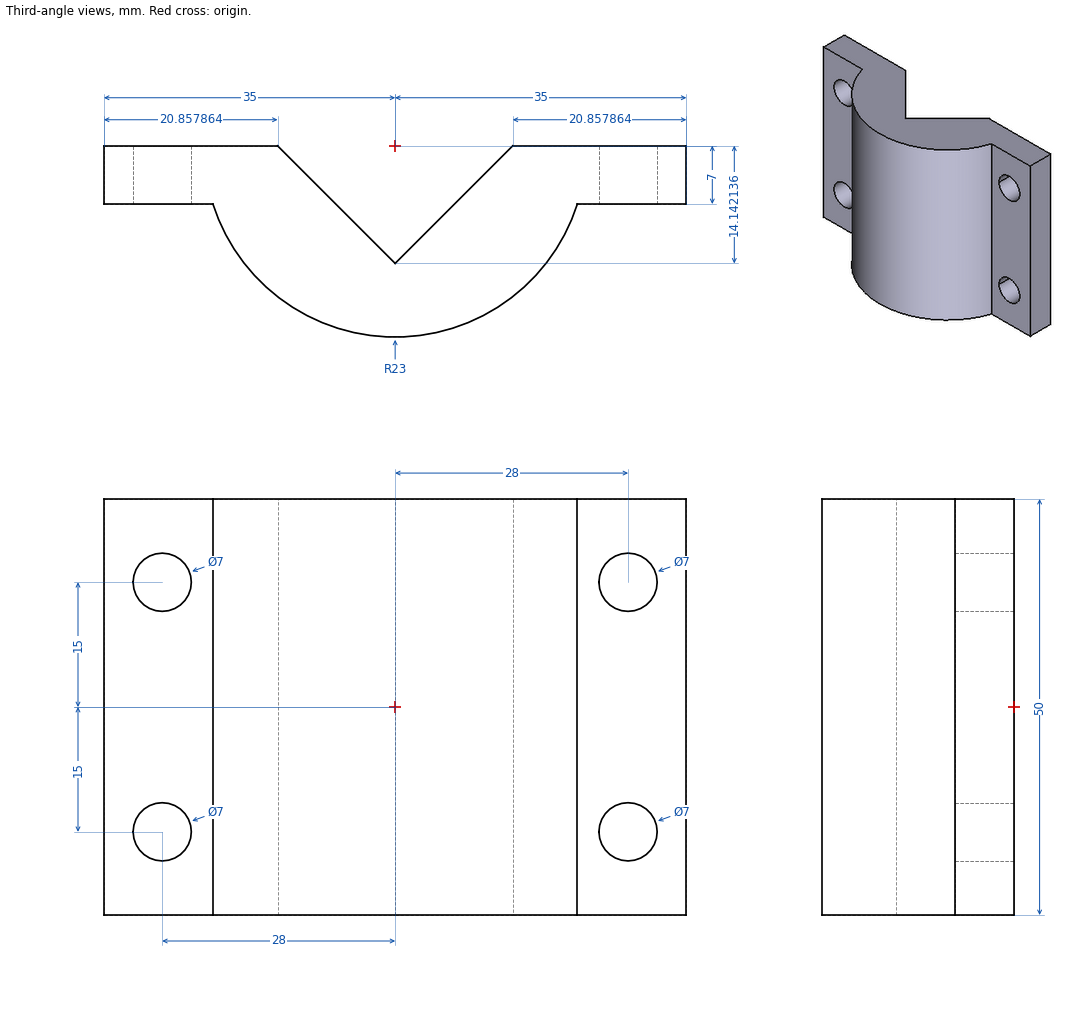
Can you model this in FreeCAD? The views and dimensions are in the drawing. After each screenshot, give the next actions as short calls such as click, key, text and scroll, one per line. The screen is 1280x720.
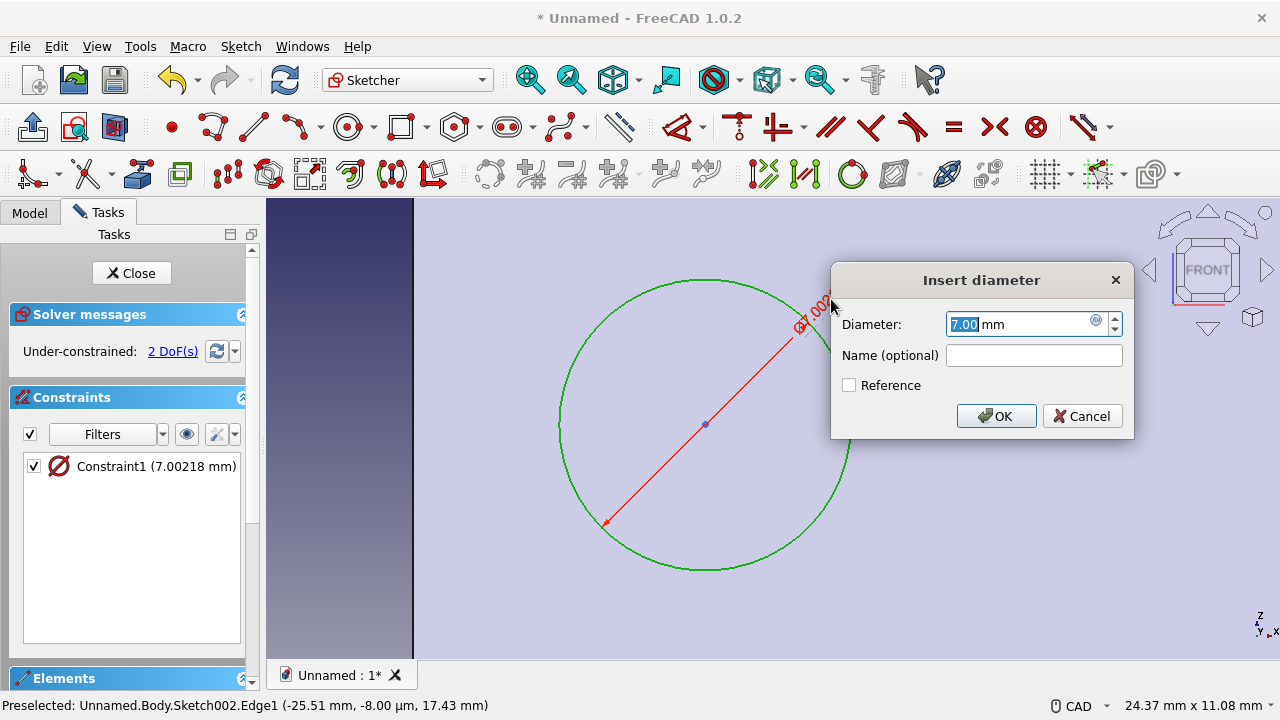
text(7)
key(Return)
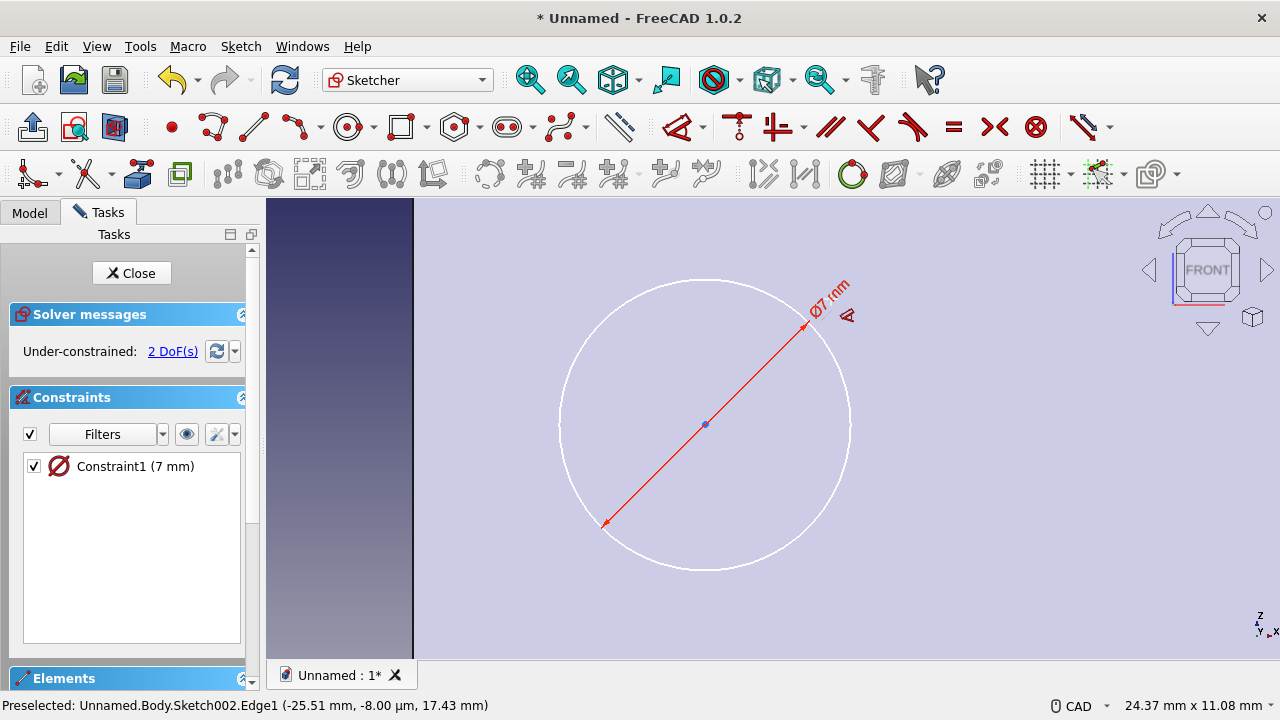
click(705, 425)
click(910, 391)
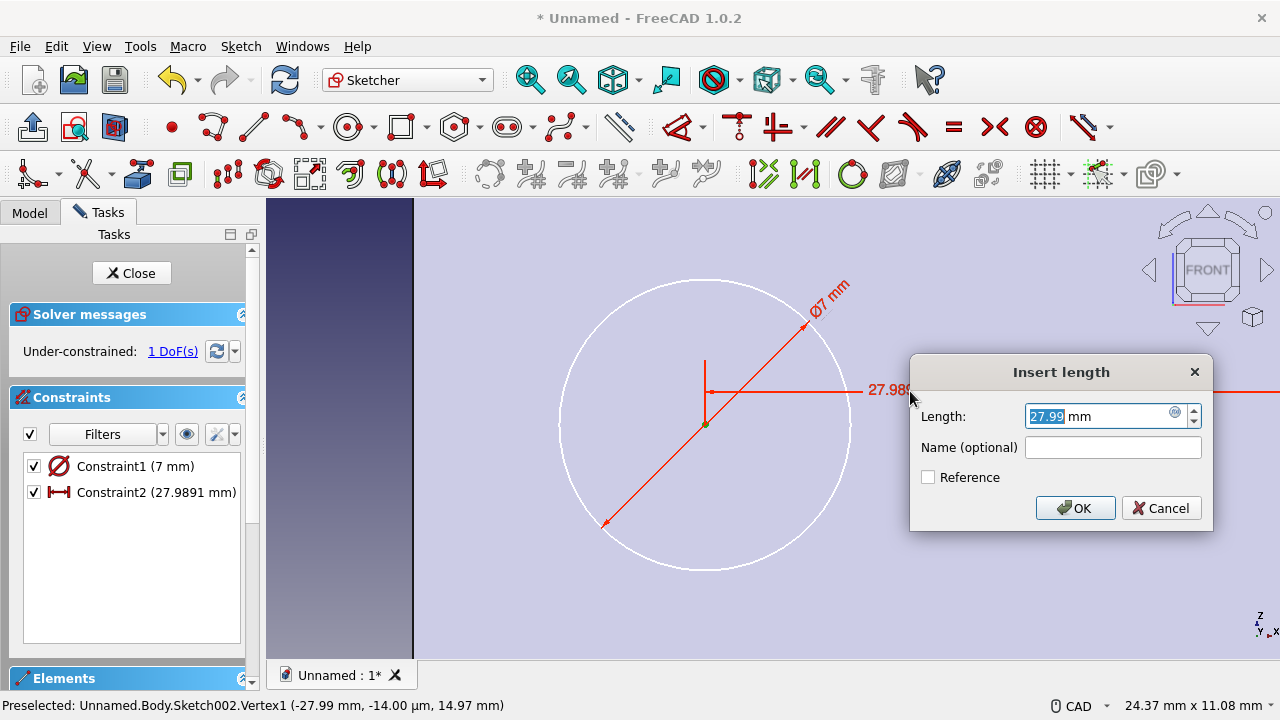
text(28)
key(Return)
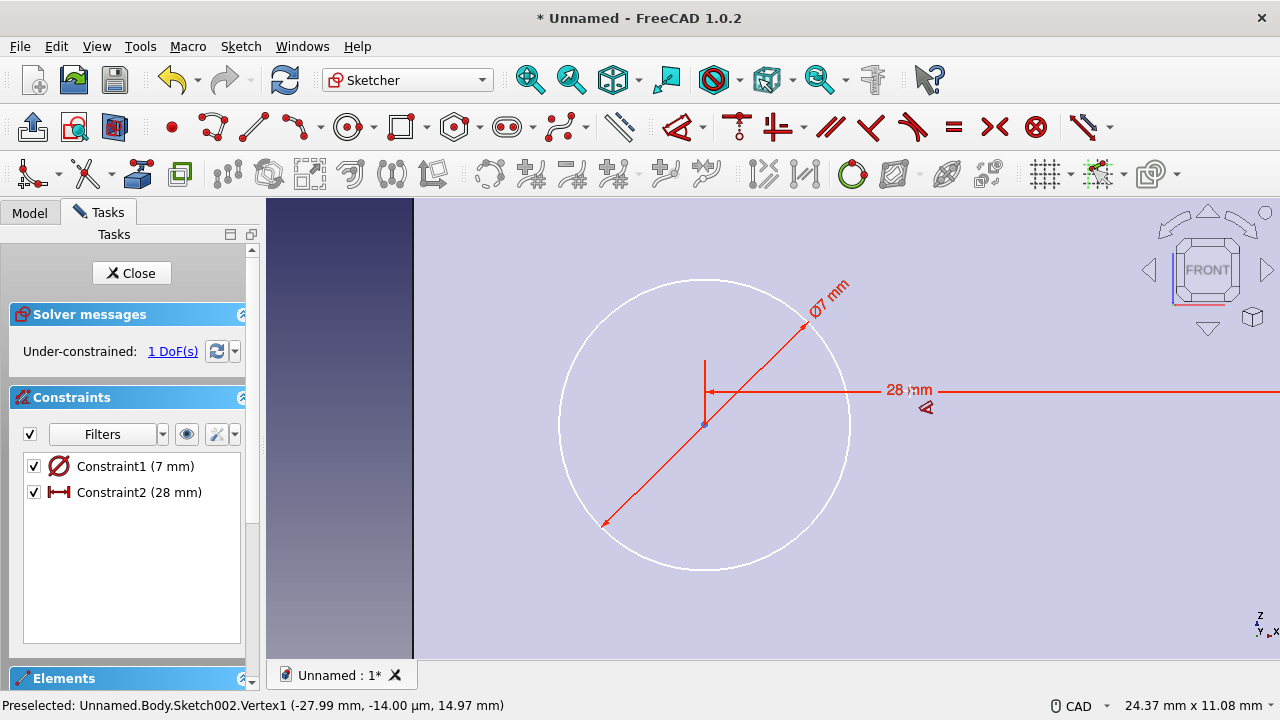
click(705, 425)
click(671, 528)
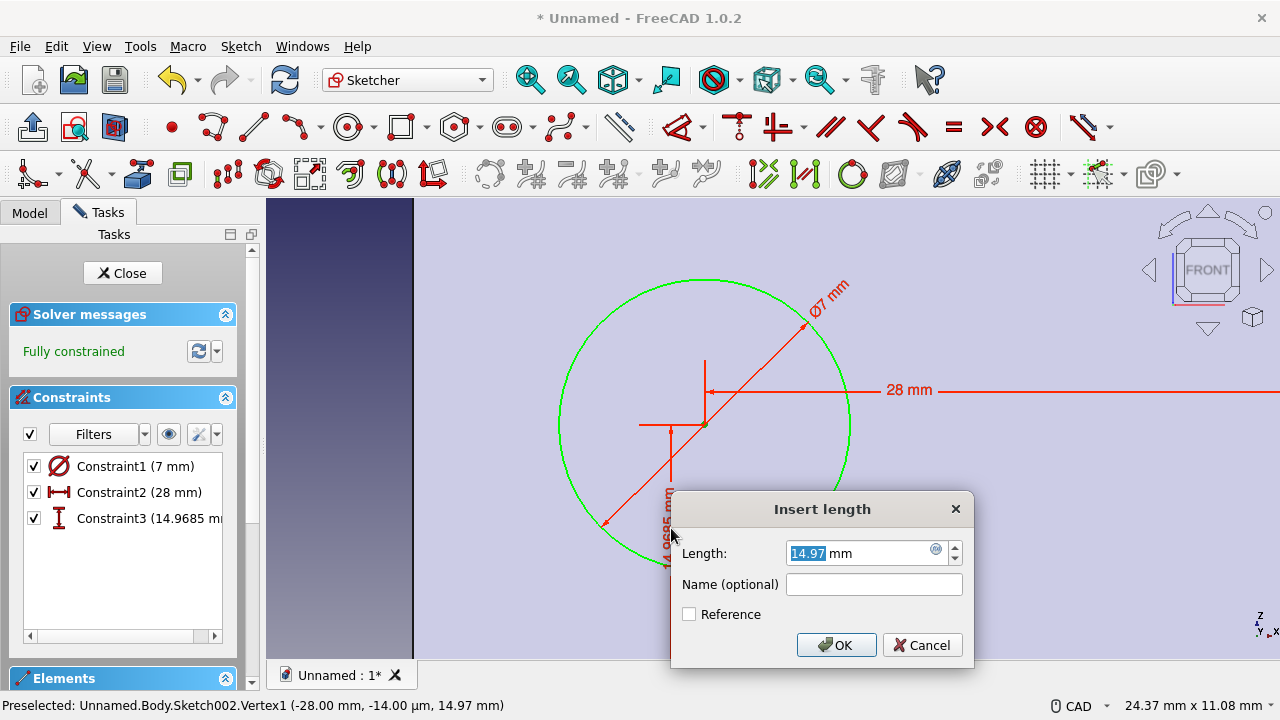
text(15)
key(Return)
key(Escape)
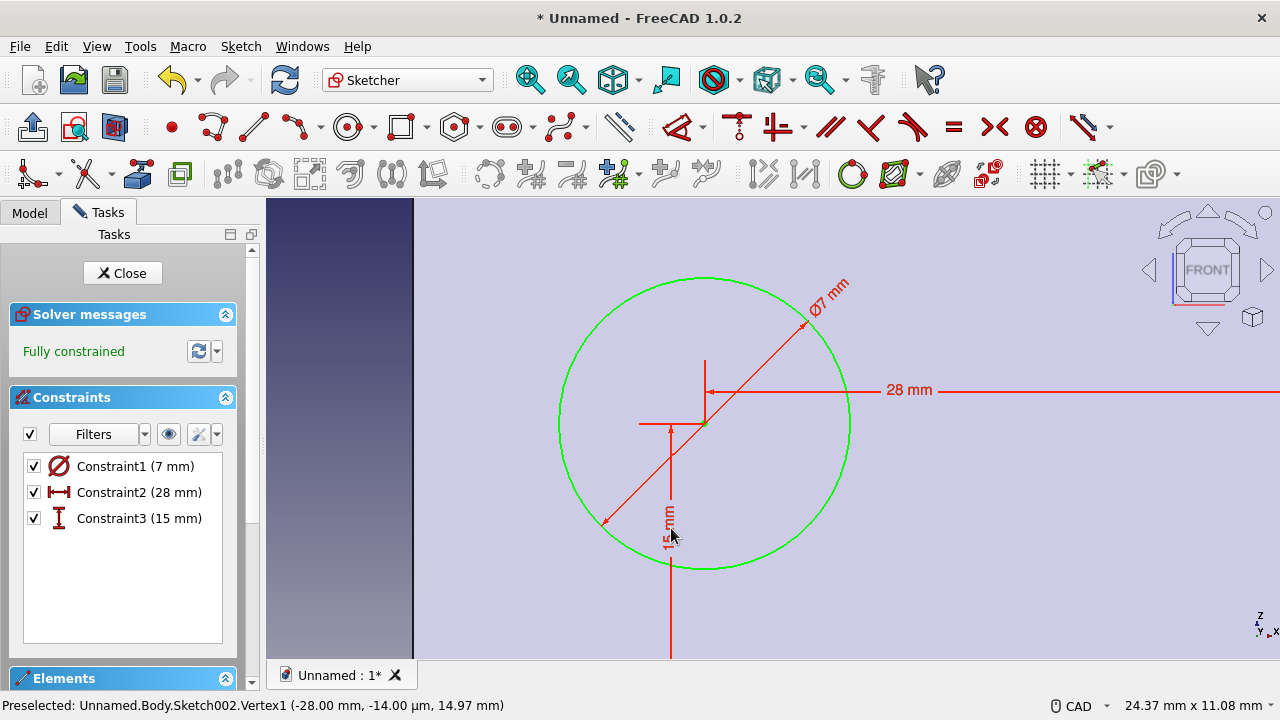
click(123, 273)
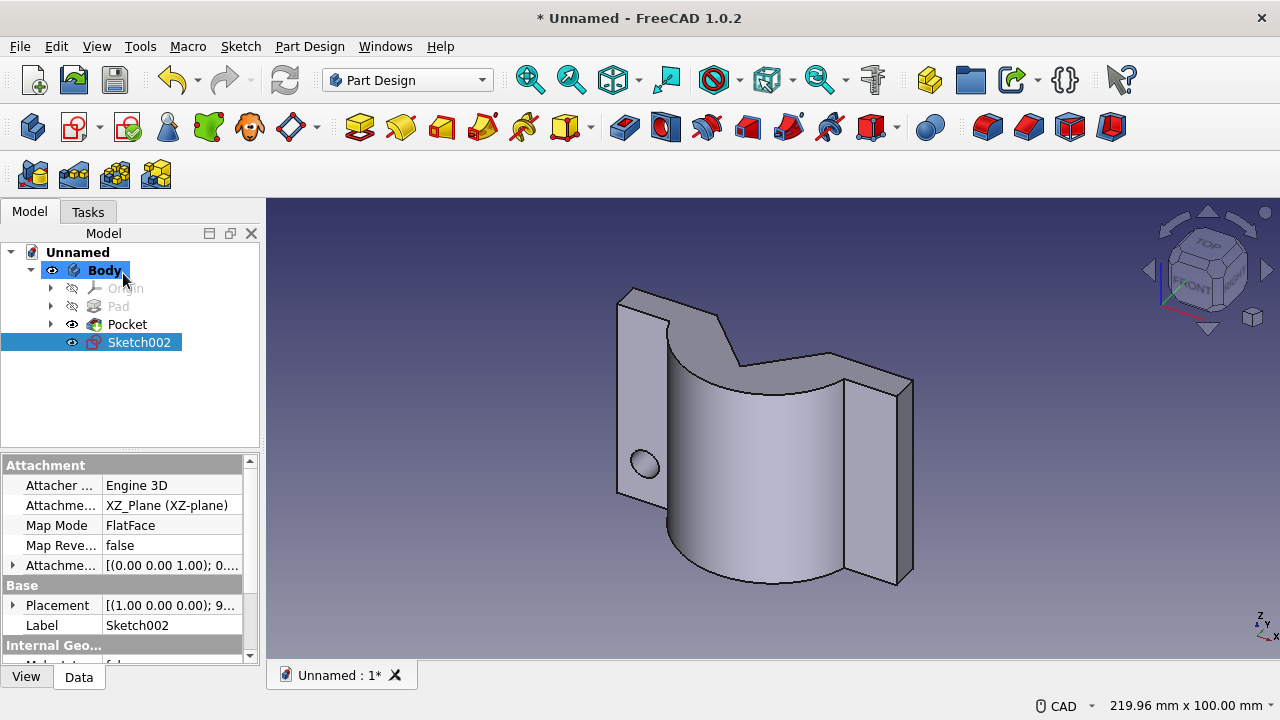
click(625, 128)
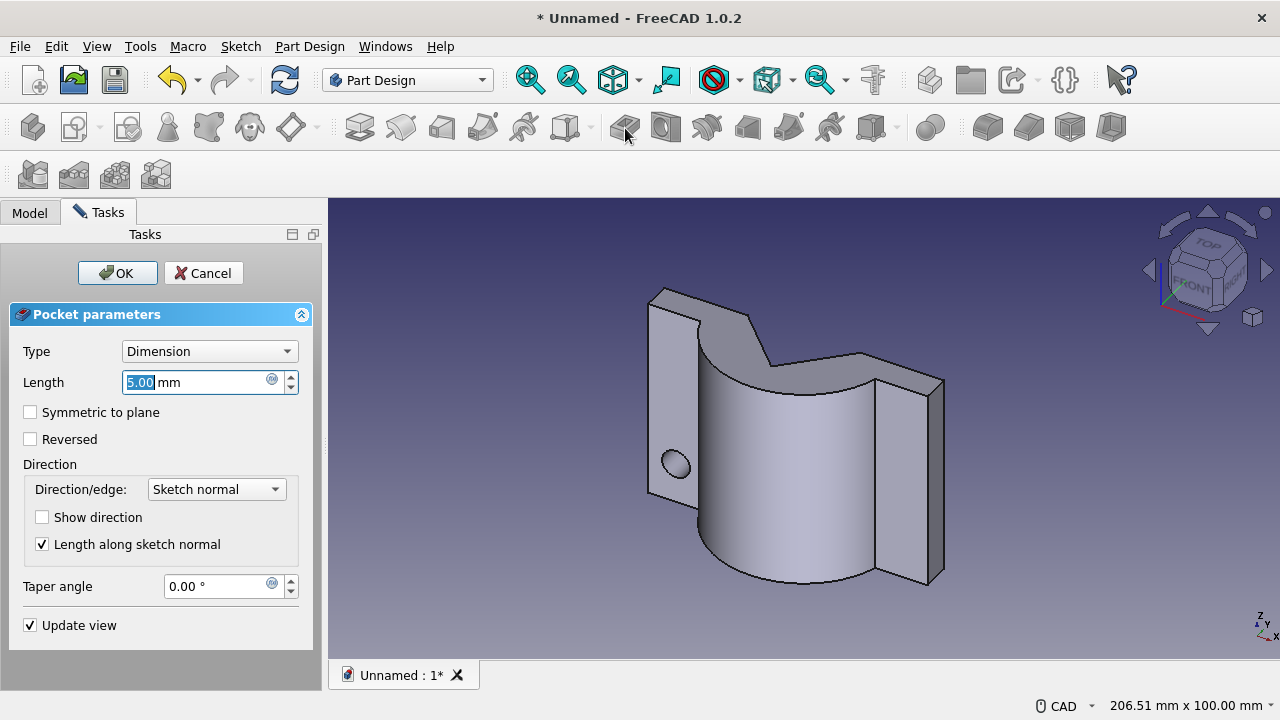
click(210, 352)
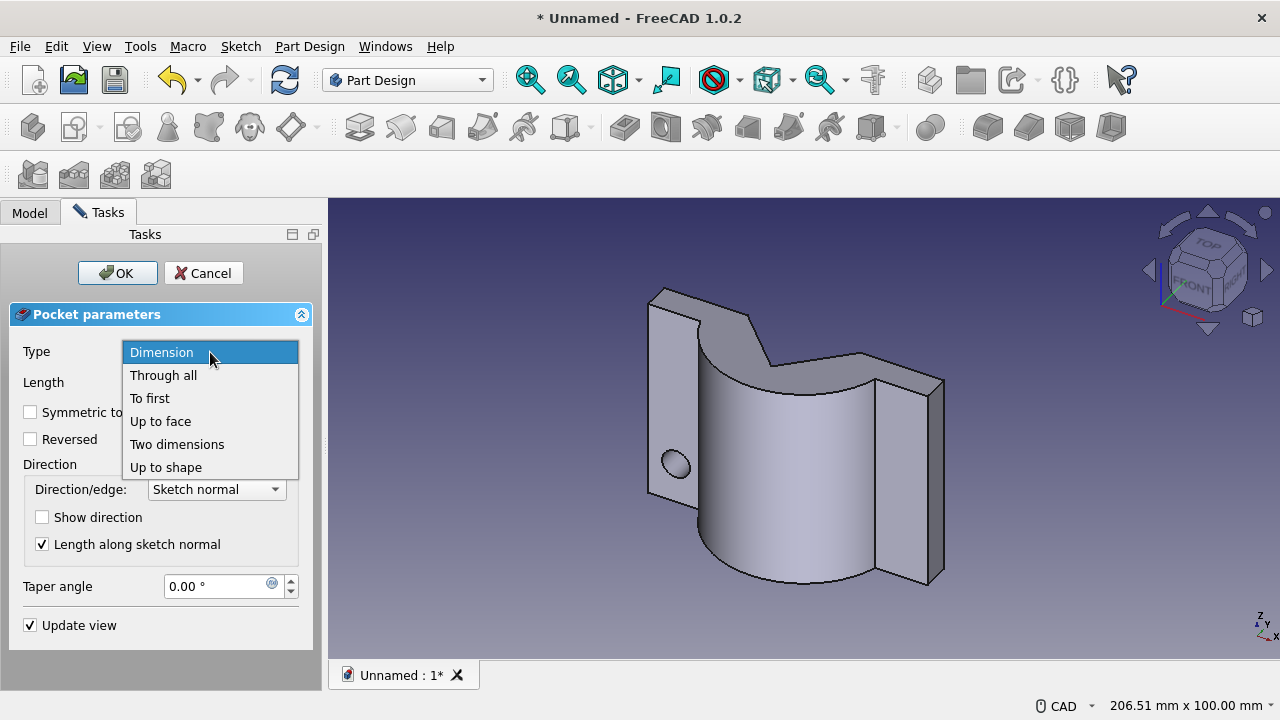
click(208, 398)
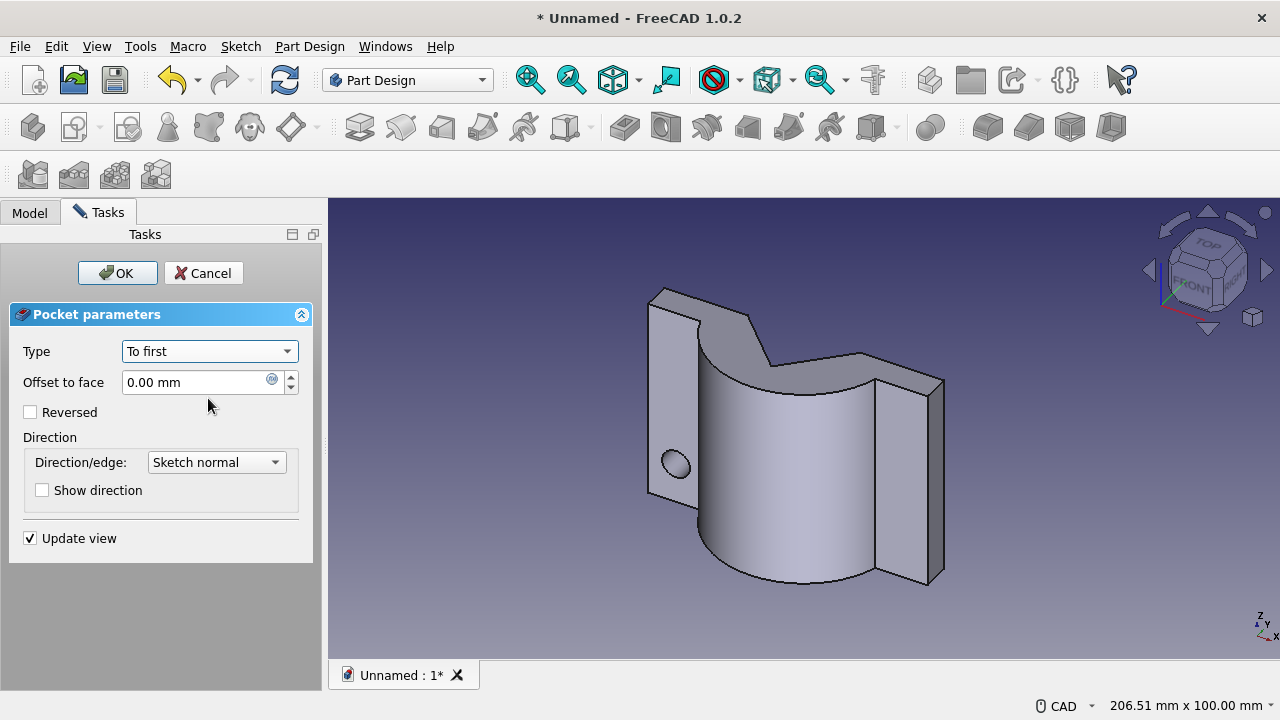
click(31, 412)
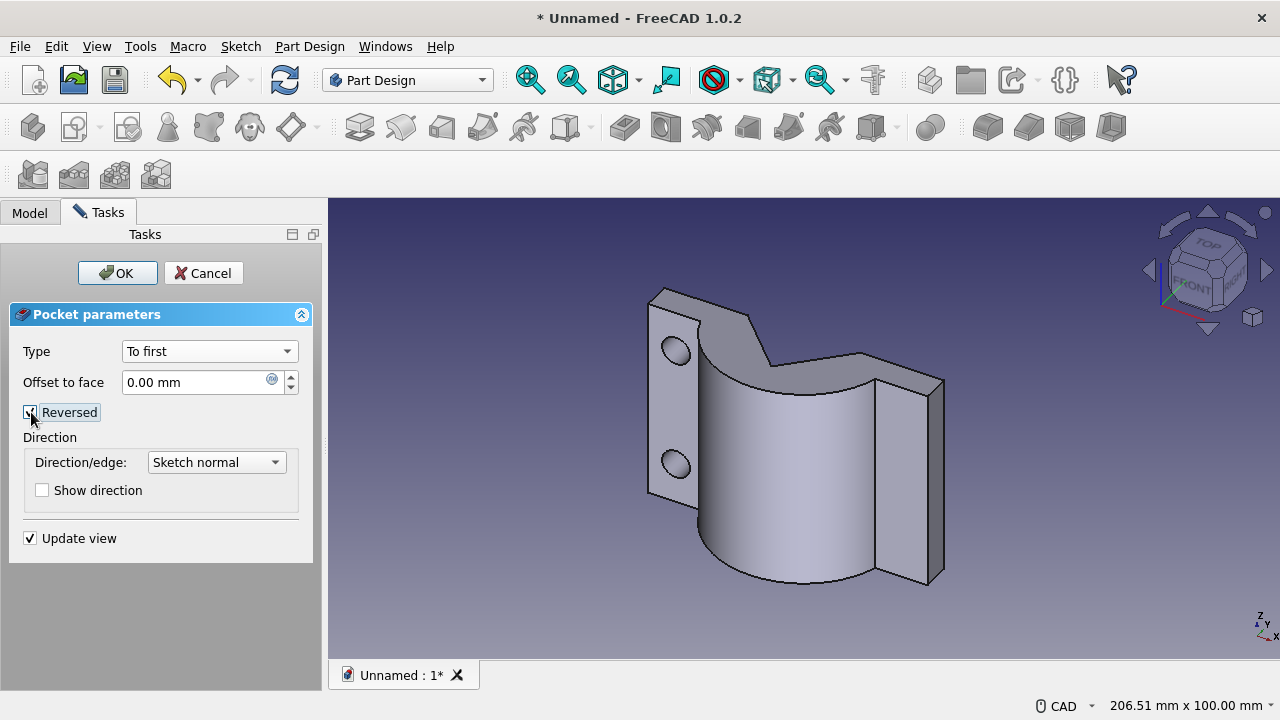
click(118, 273)